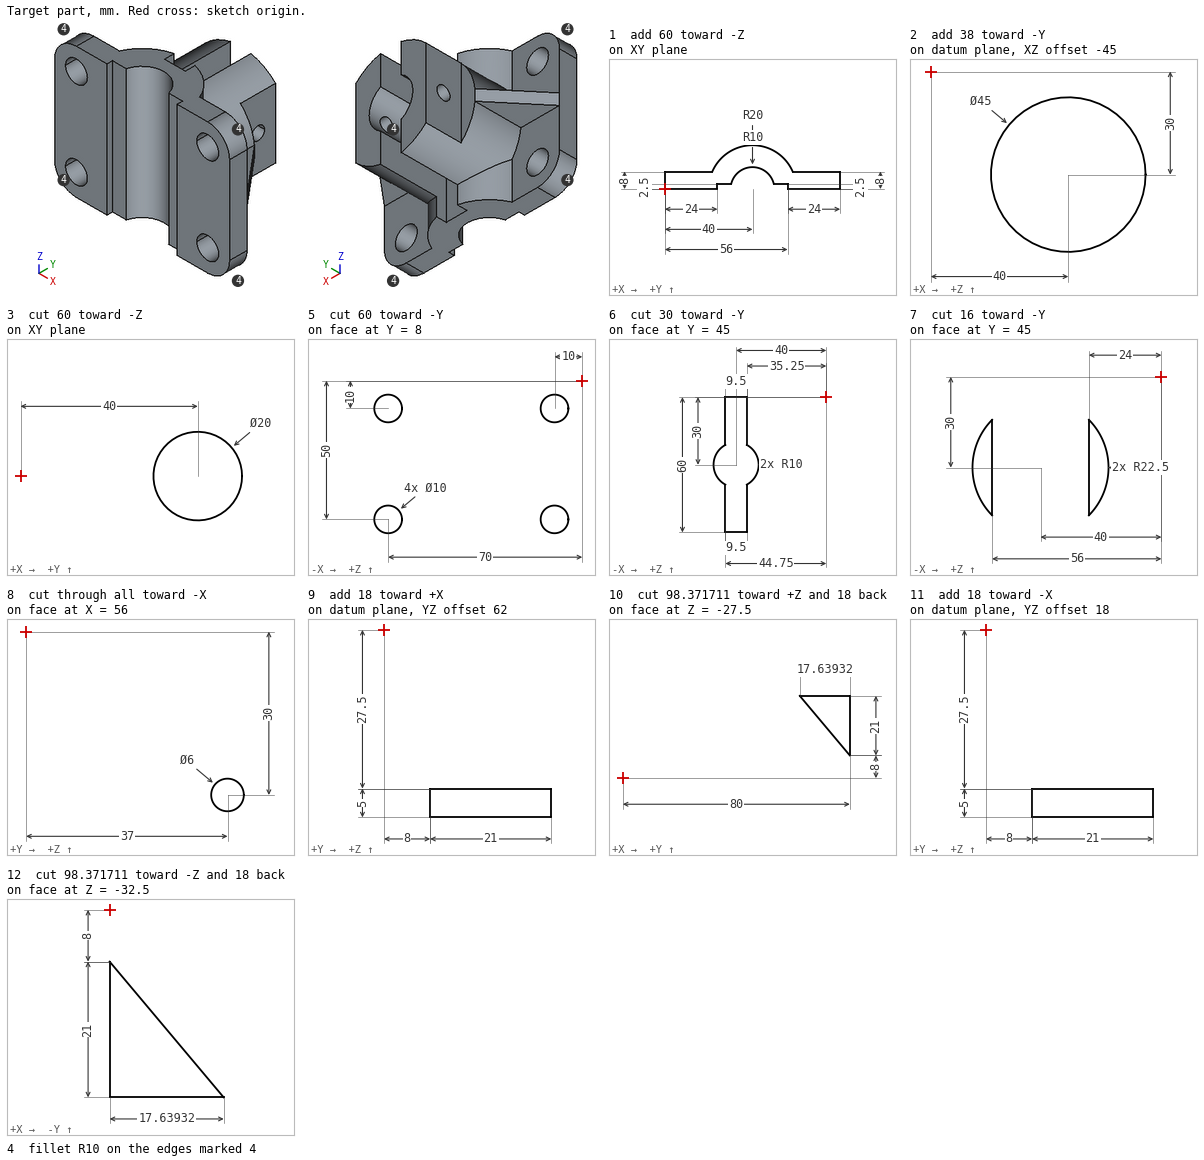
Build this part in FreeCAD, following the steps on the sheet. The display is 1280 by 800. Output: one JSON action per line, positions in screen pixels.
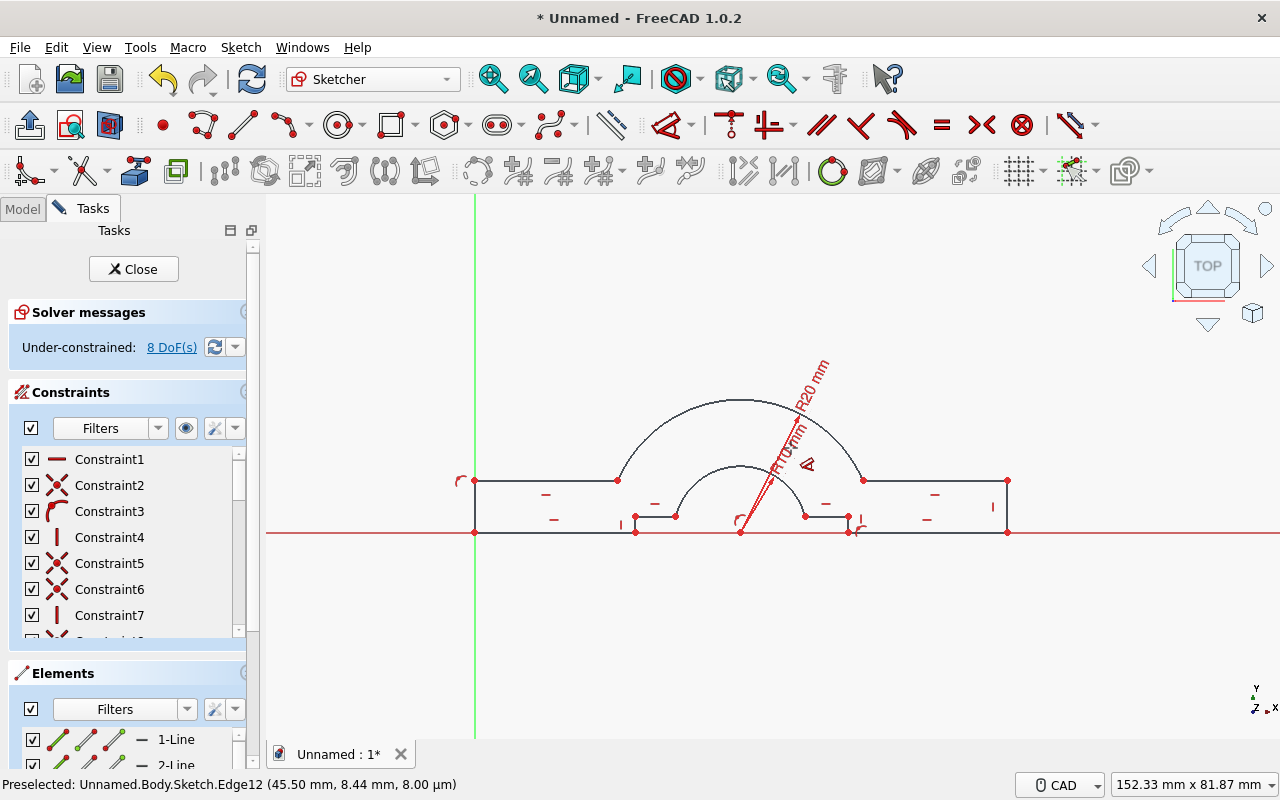
{"action": "left_click", "coordinate": [1007, 517]}
{"action": "left_click", "coordinate": [1041, 507]}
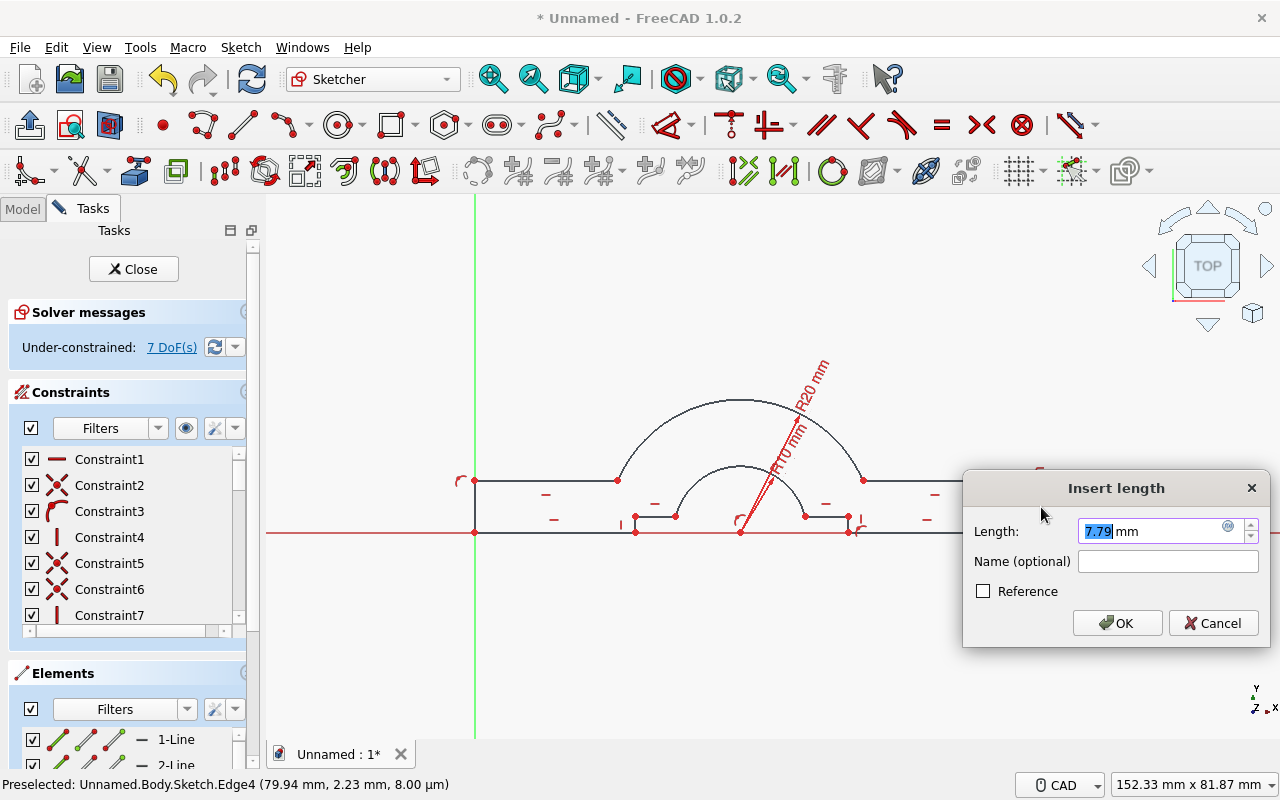
{"action": "type", "text": "8"}
{"action": "key", "text": "Return"}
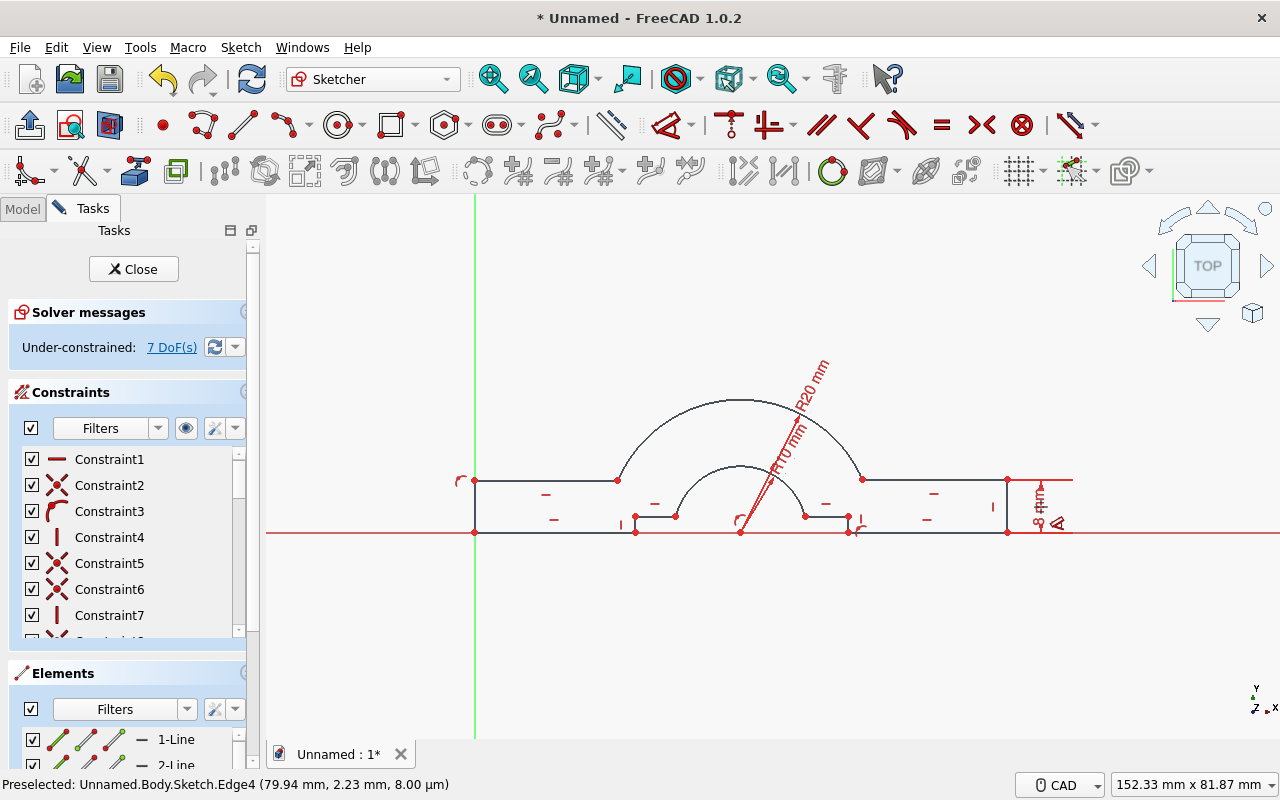
{"action": "left_click", "coordinate": [475, 497]}
{"action": "left_click", "coordinate": [441, 507]}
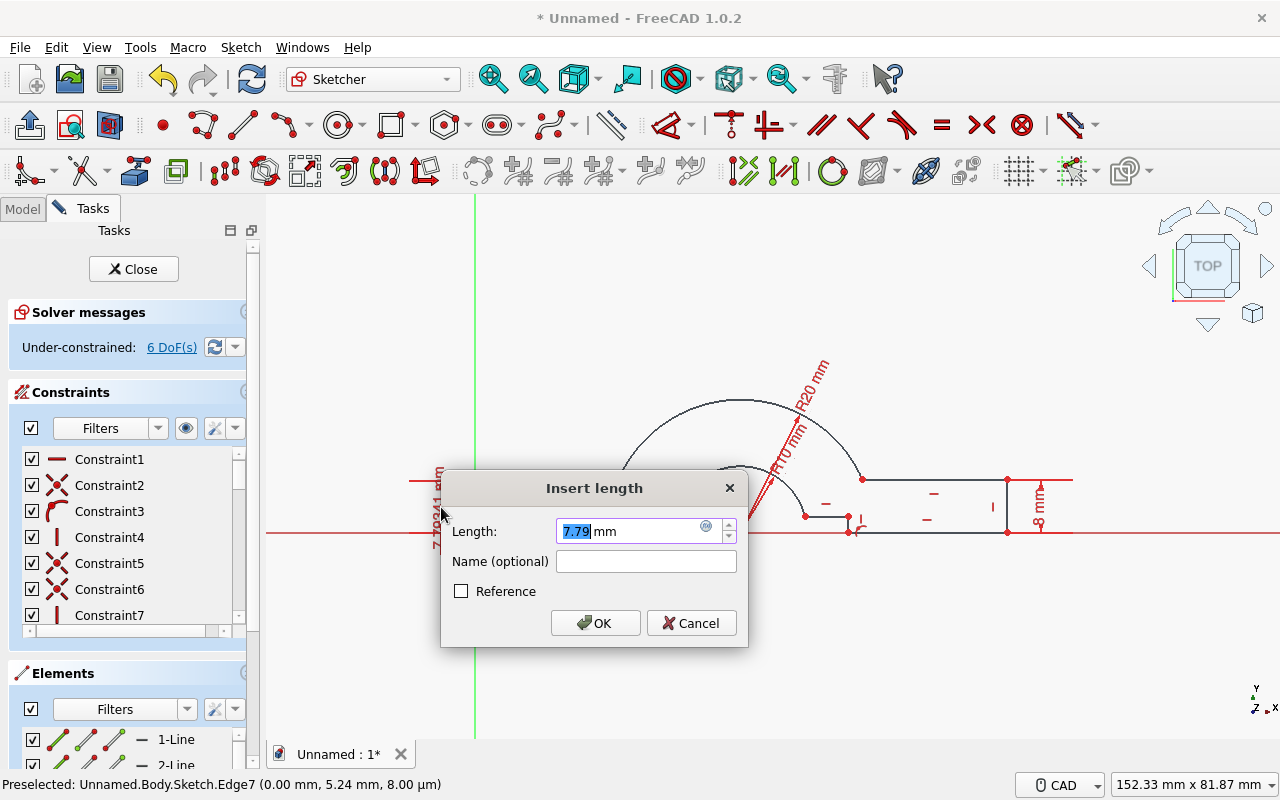
{"action": "type", "text": "8"}
{"action": "key", "text": "Return"}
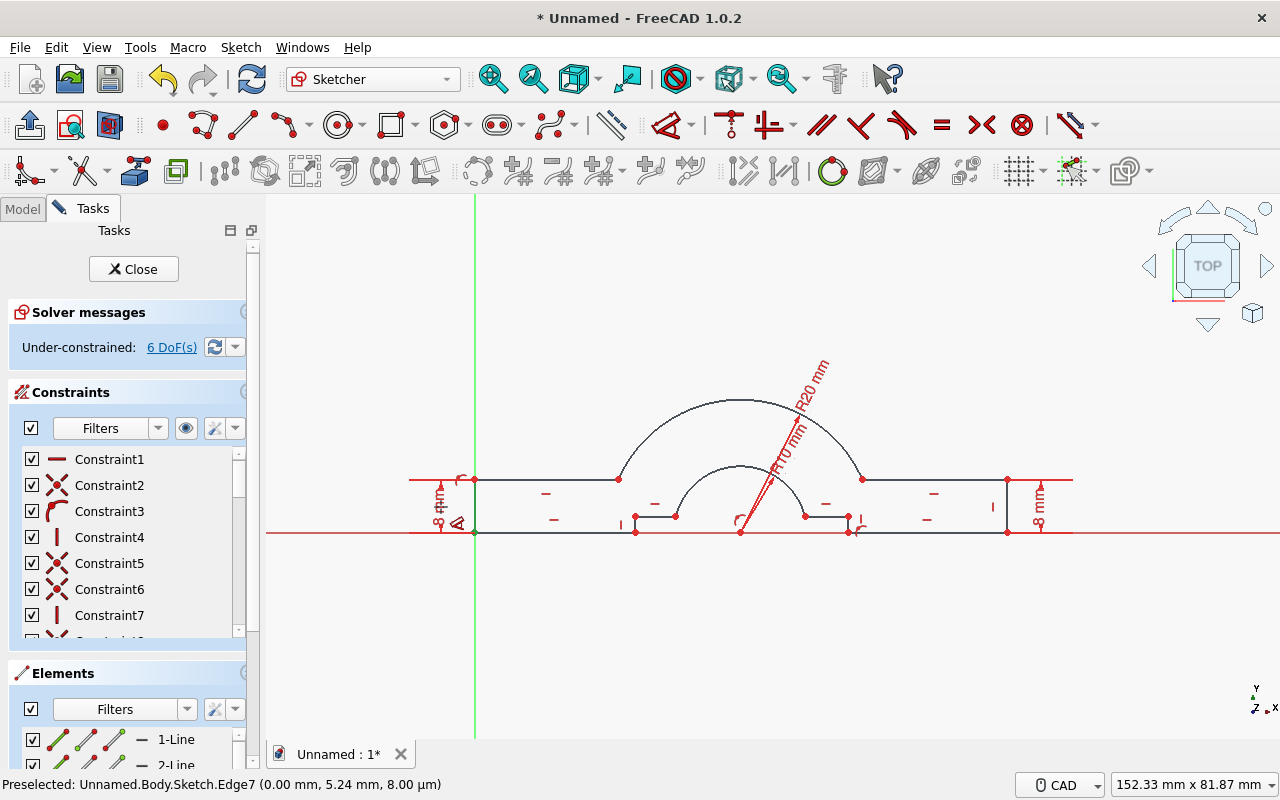
{"action": "left_click", "coordinate": [896, 533]}
{"action": "left_click", "coordinate": [927, 567]}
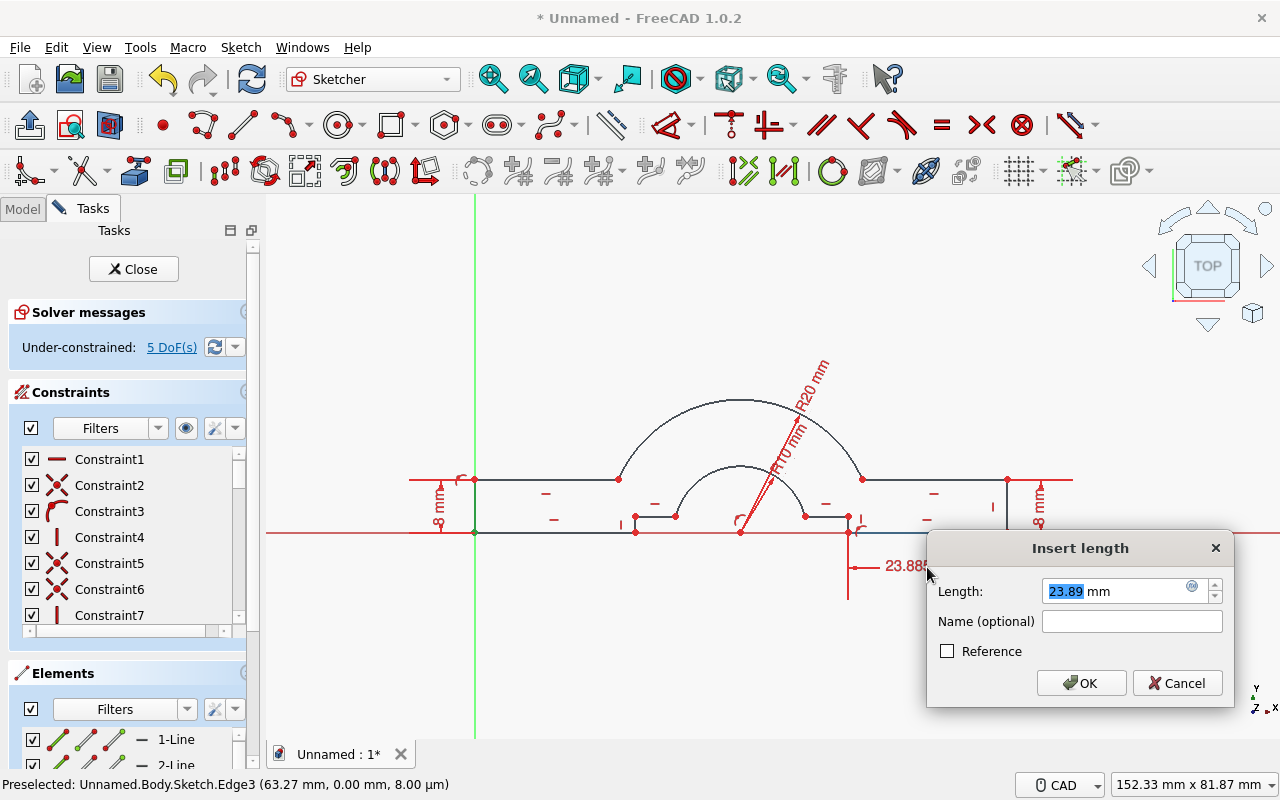
{"action": "type", "text": "24"}
{"action": "key", "text": "Return"}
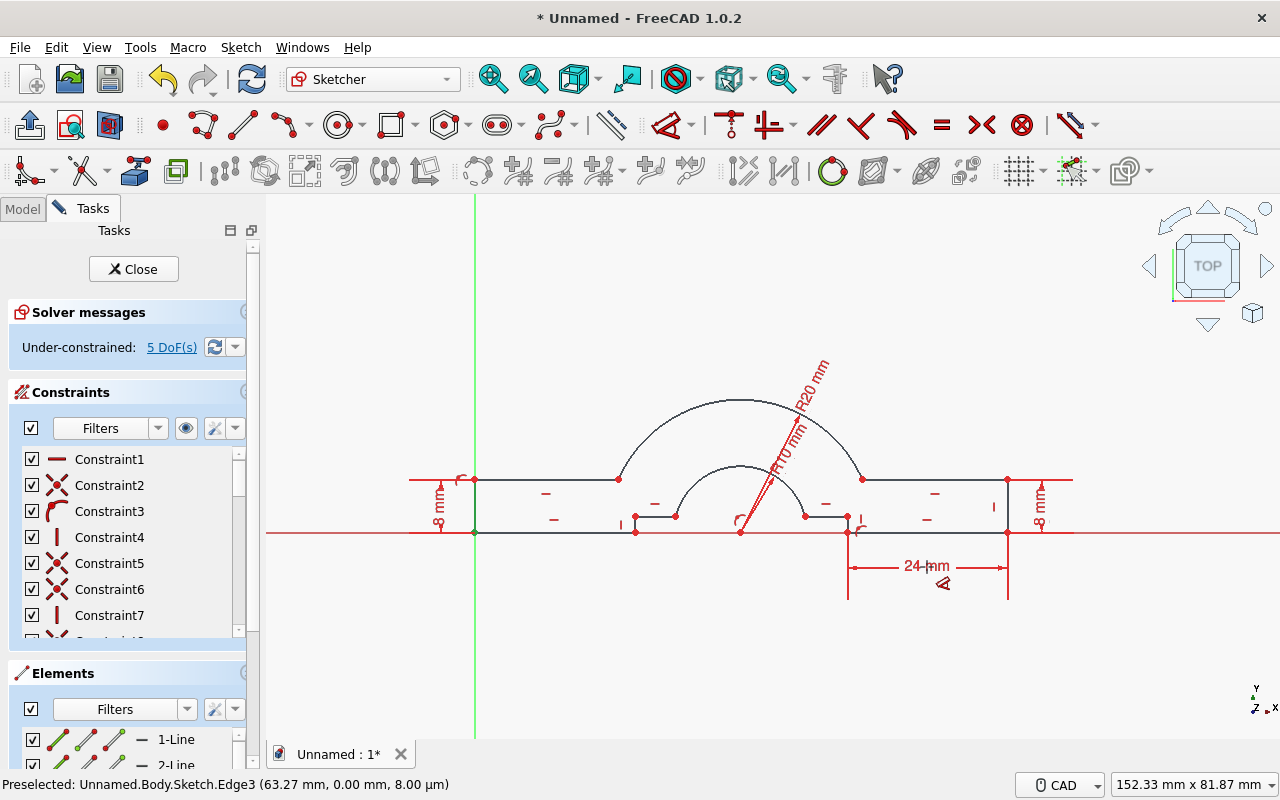
{"action": "left_click", "coordinate": [523, 533]}
{"action": "left_click", "coordinate": [555, 567]}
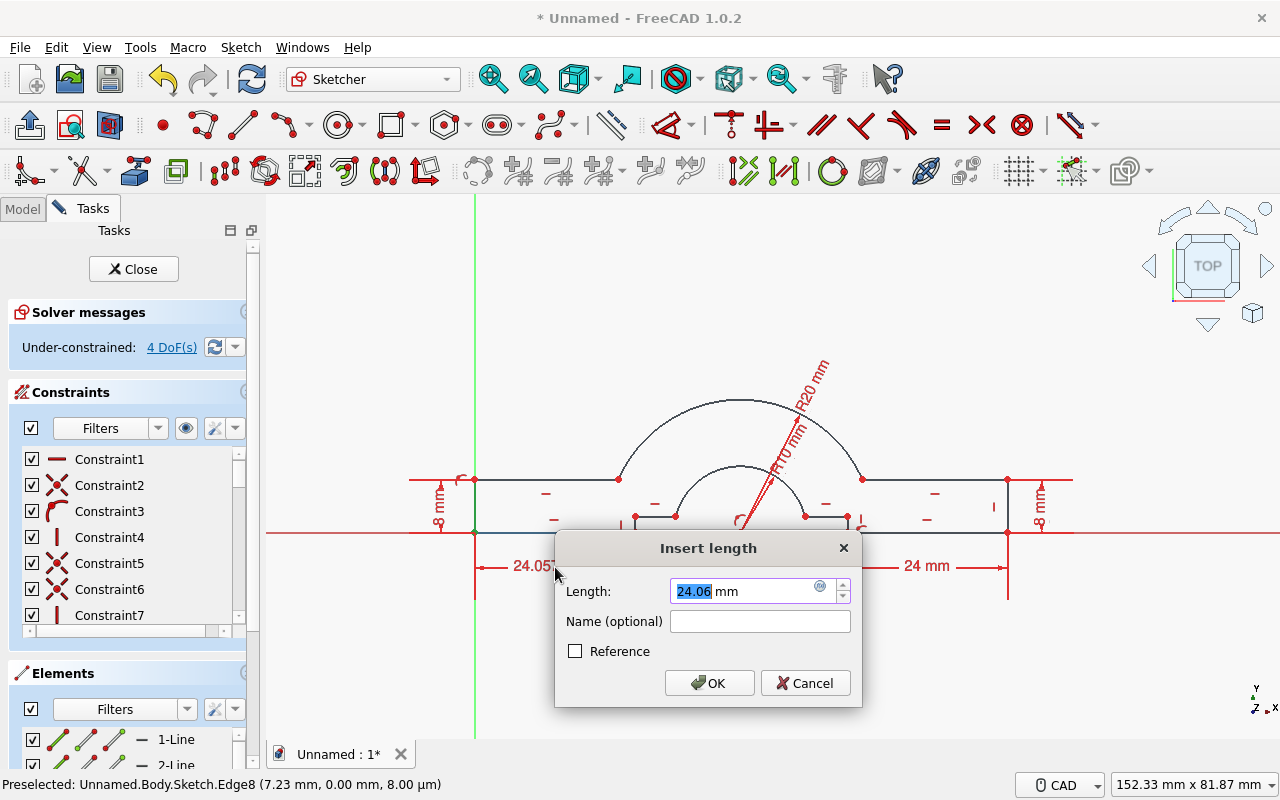
{"action": "type", "text": "24"}
{"action": "key", "text": "Return"}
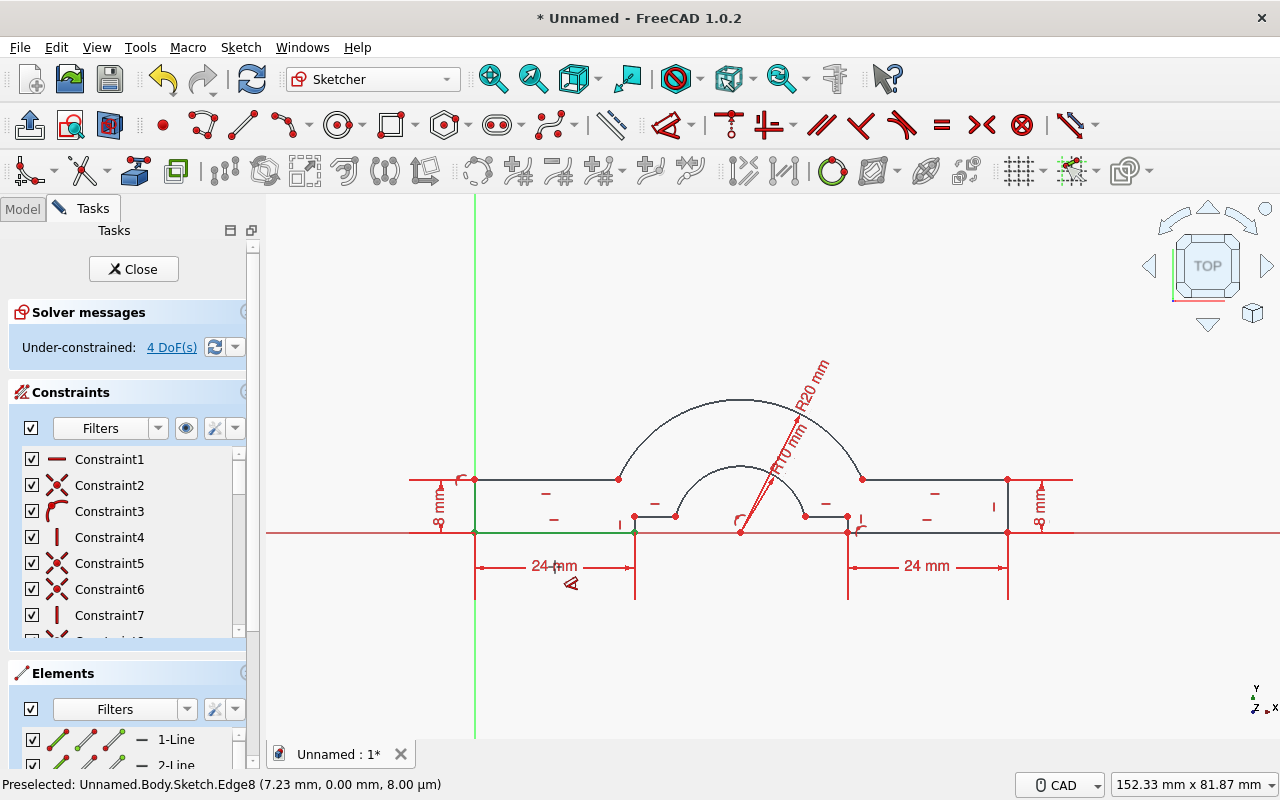
{"action": "scroll", "coordinate": [848, 525], "scroll_direction": "up", "scroll_amount": 5}